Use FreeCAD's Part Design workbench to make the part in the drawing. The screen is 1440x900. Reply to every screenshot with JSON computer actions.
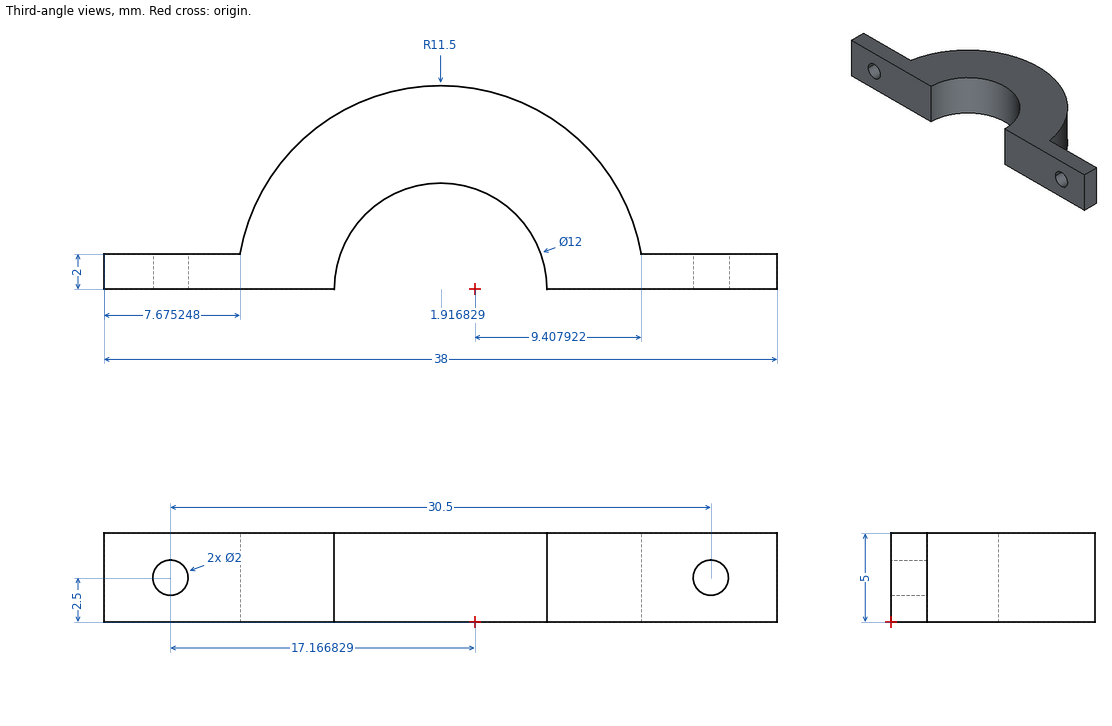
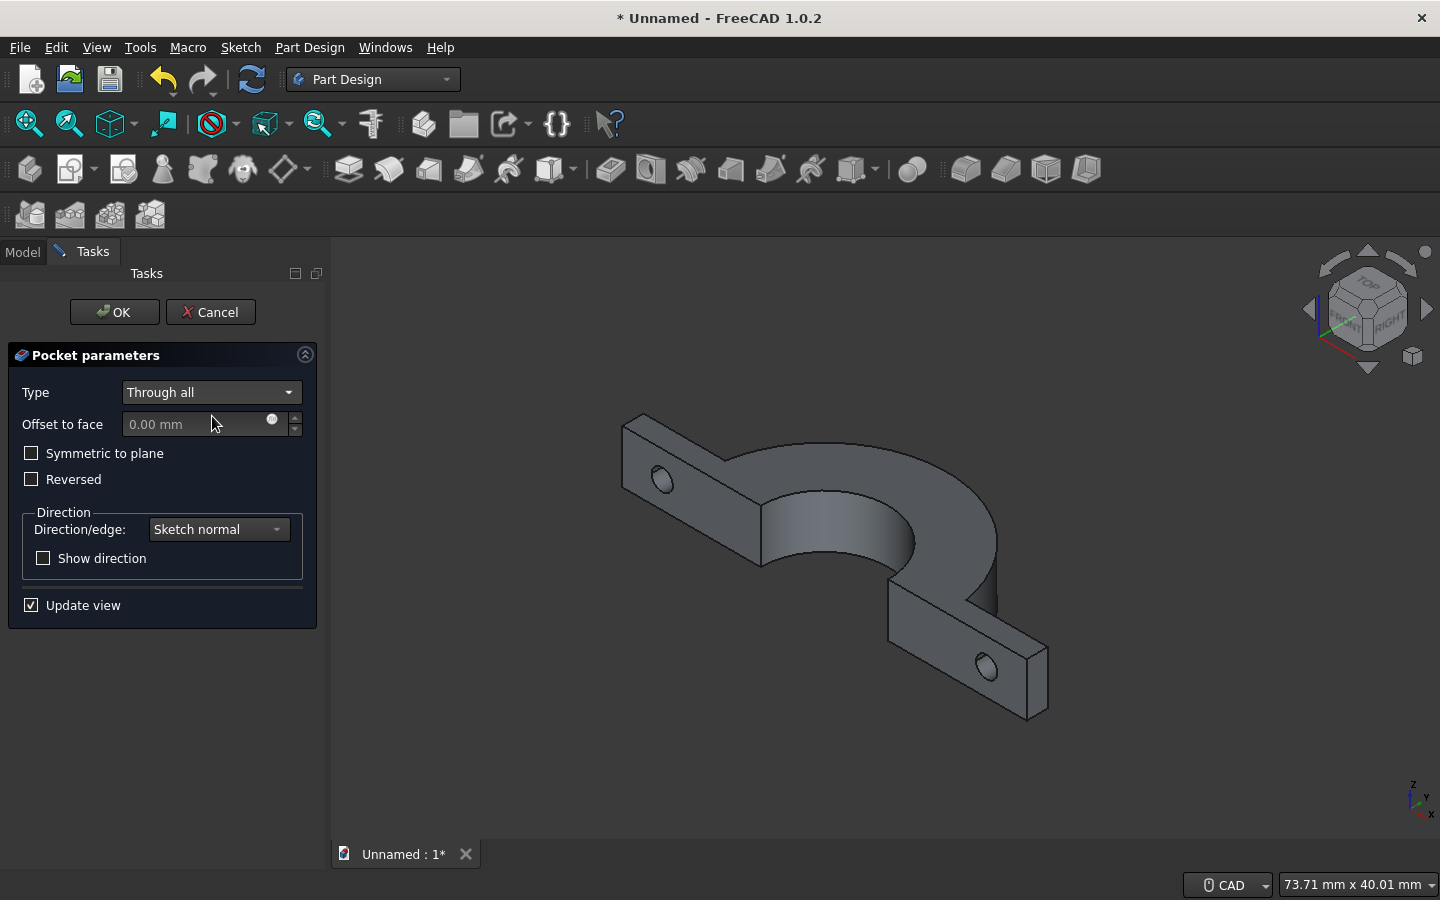
{"action": "left_click", "coordinate": [115, 312]}